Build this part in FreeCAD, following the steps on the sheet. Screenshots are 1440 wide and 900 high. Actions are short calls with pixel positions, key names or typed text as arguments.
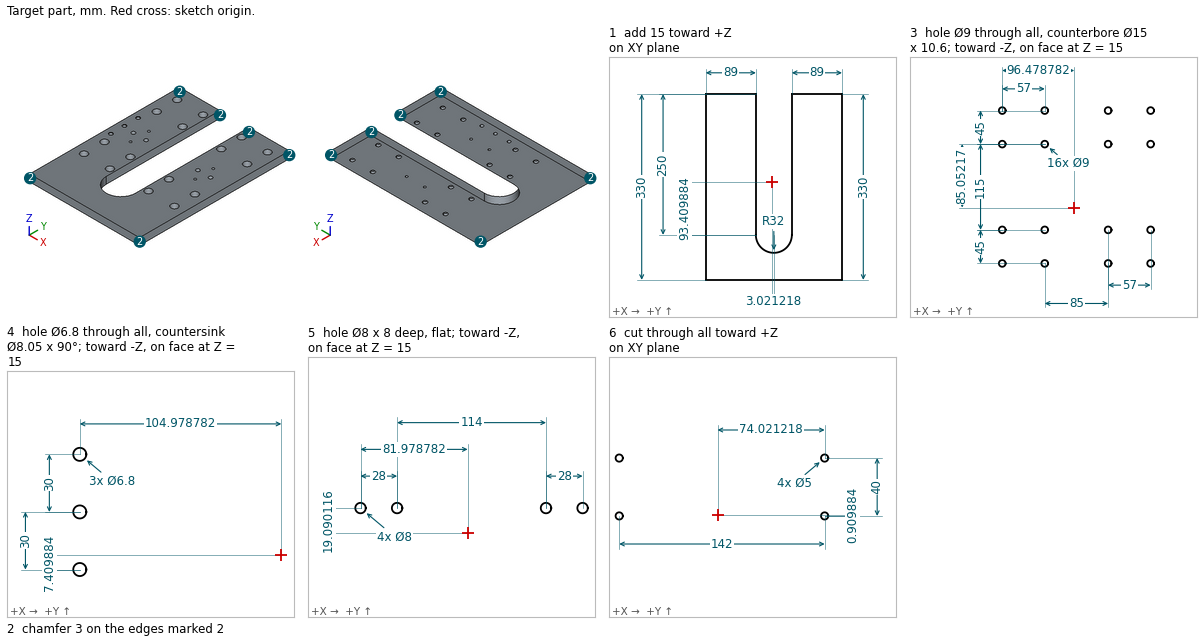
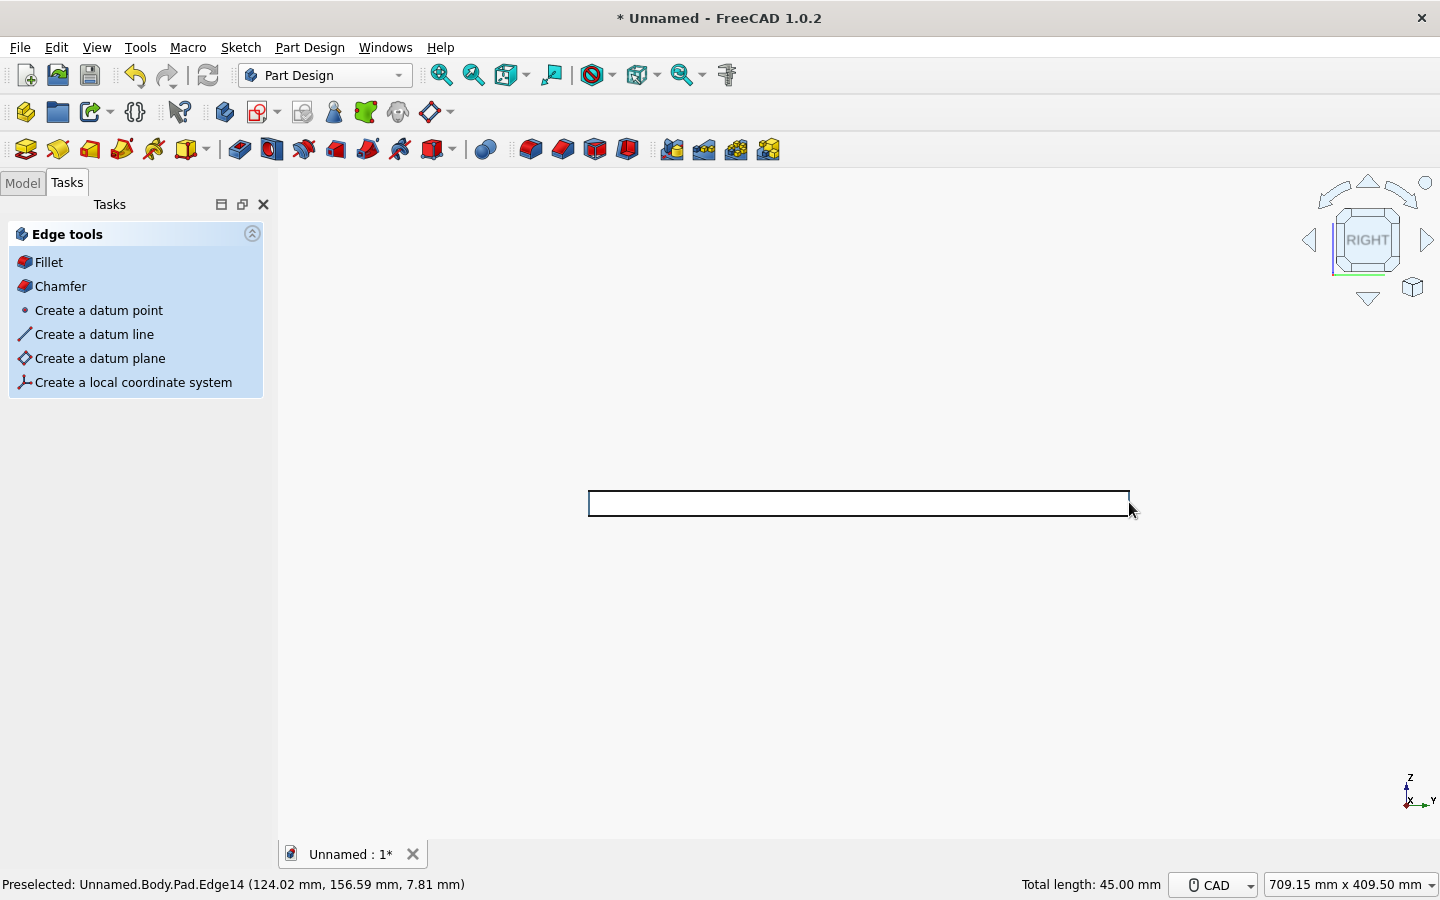
key(5)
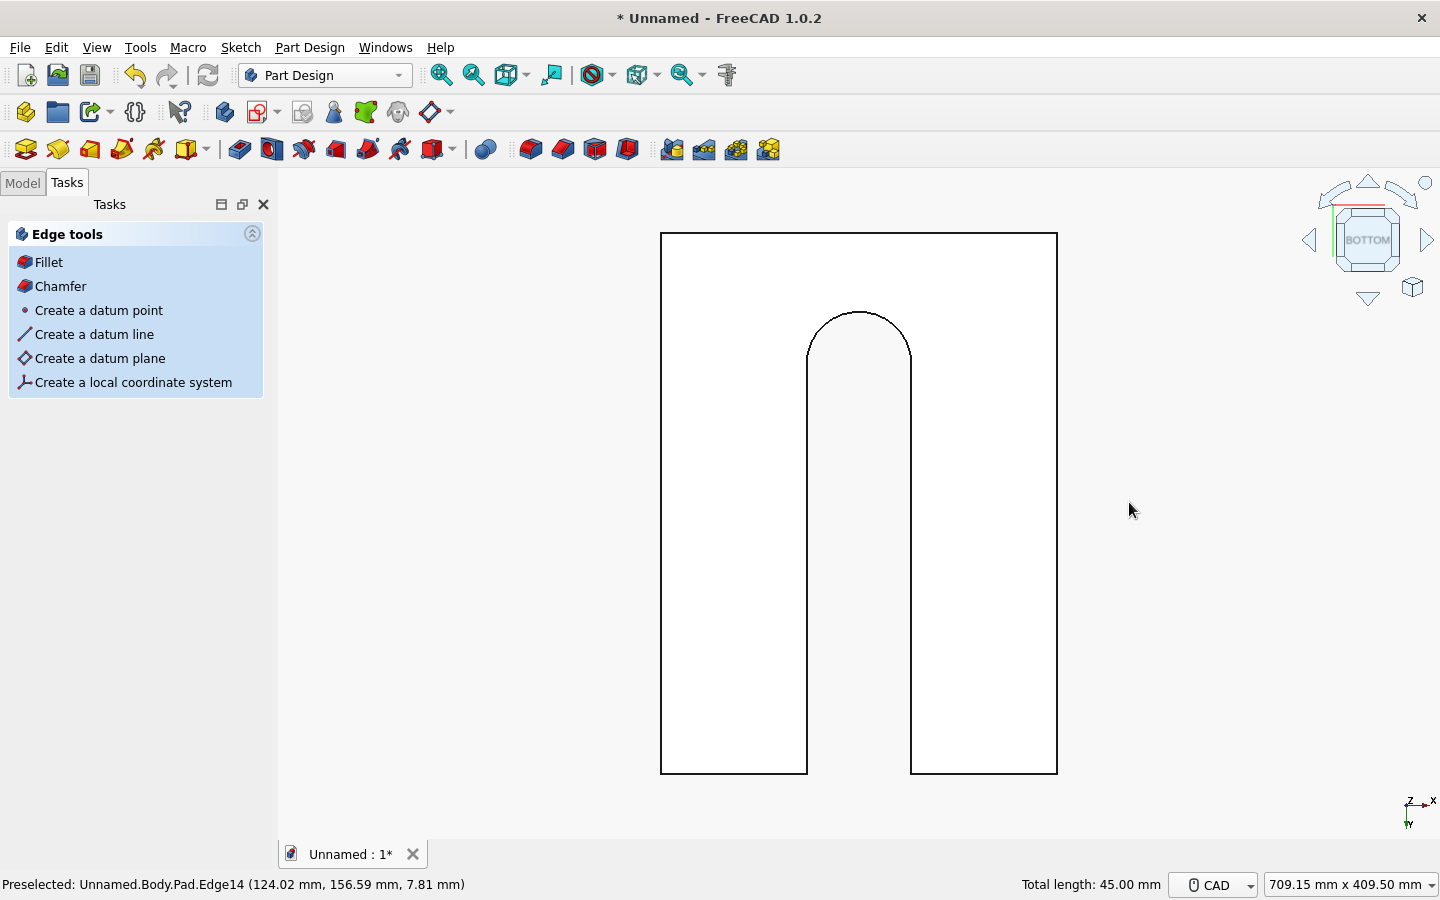
key(4)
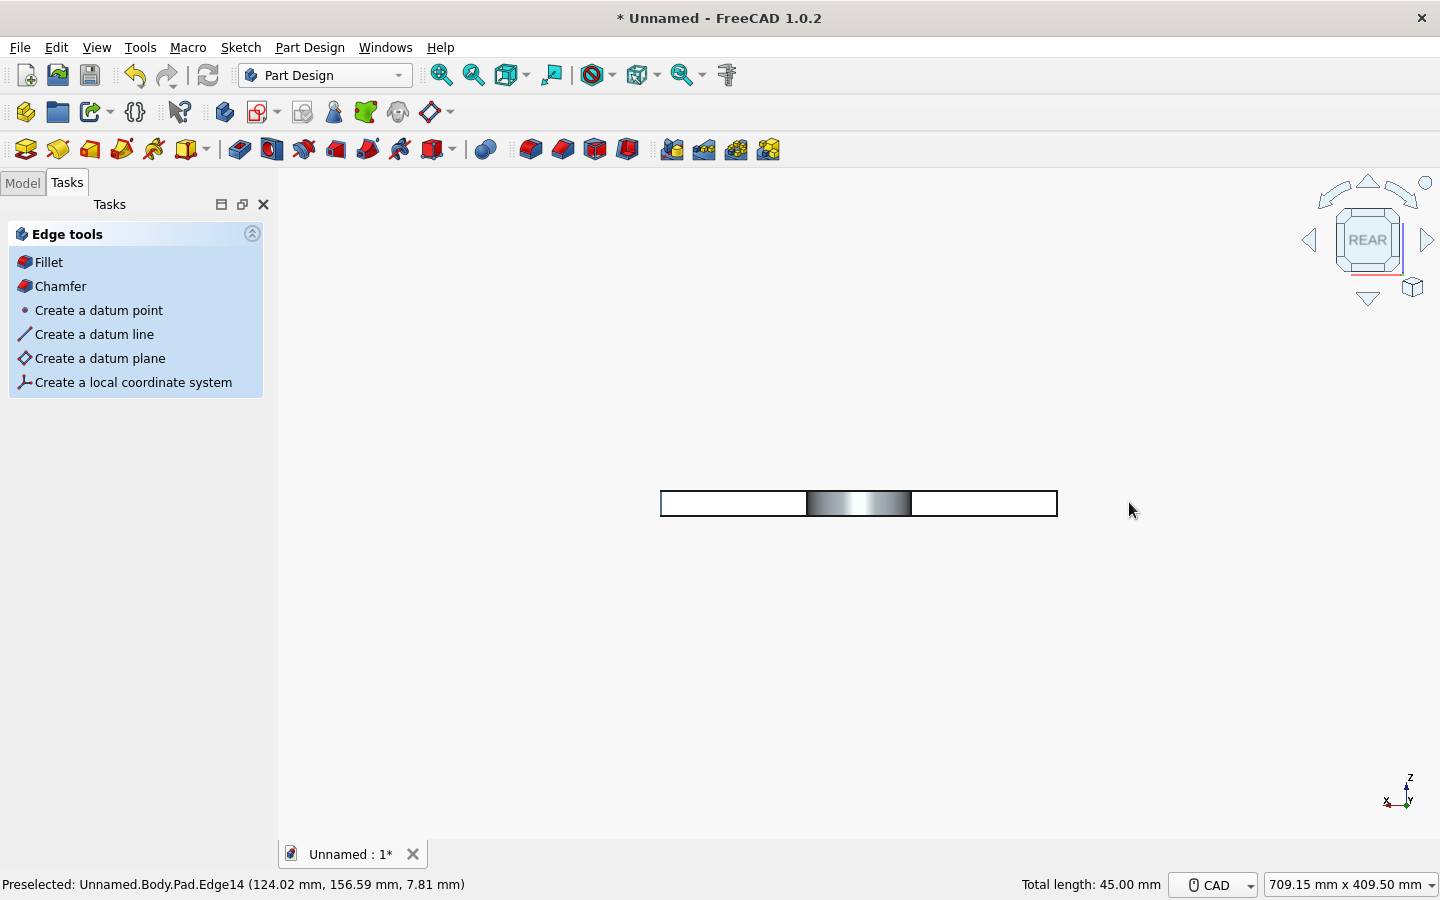
click(442, 76)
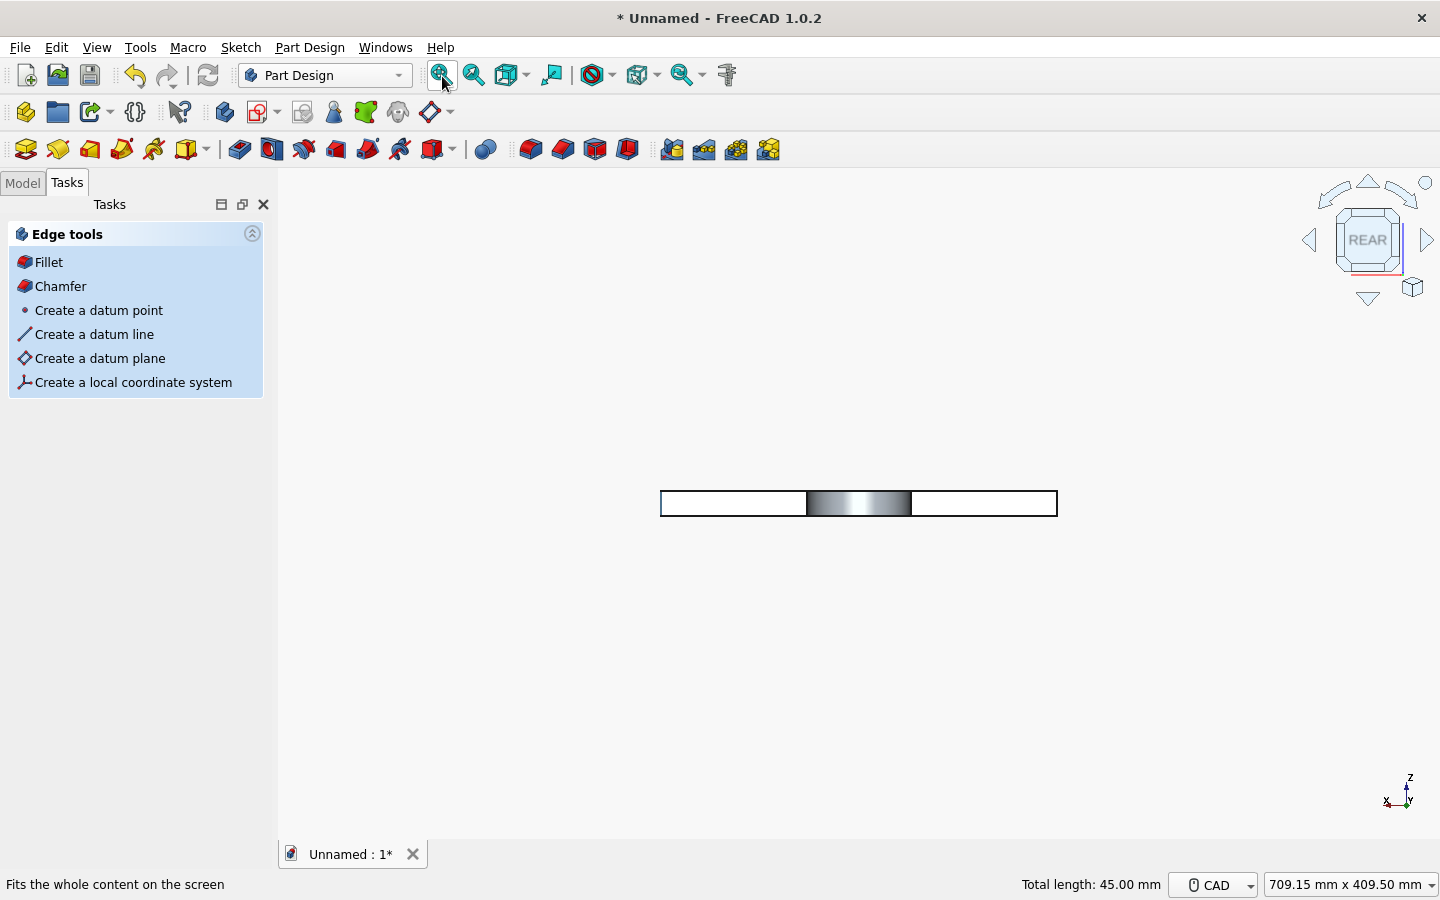
click(1057, 503, ctrl)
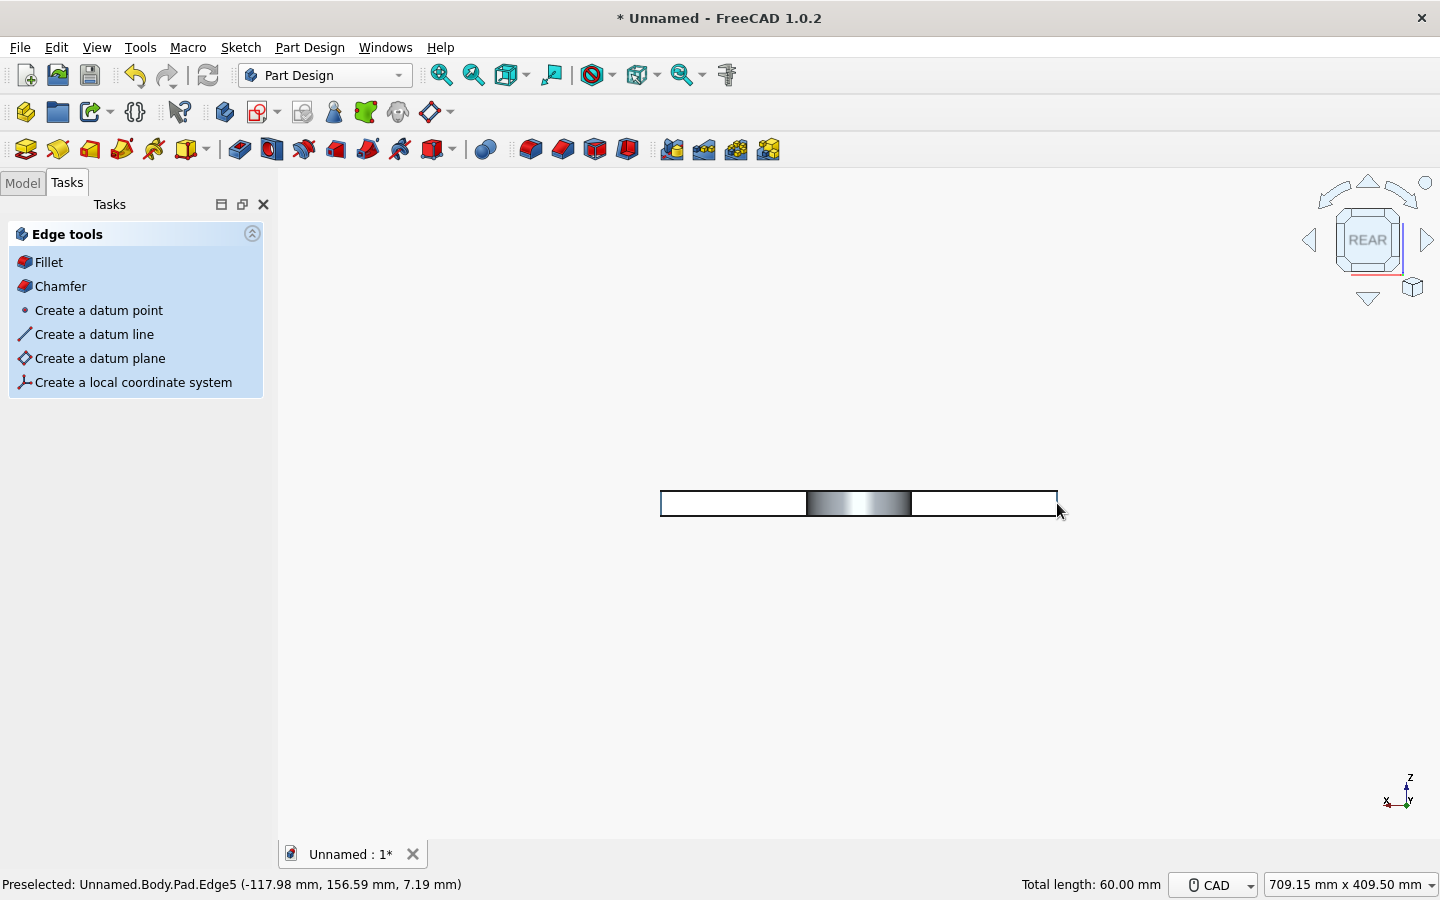
click(911, 503, ctrl)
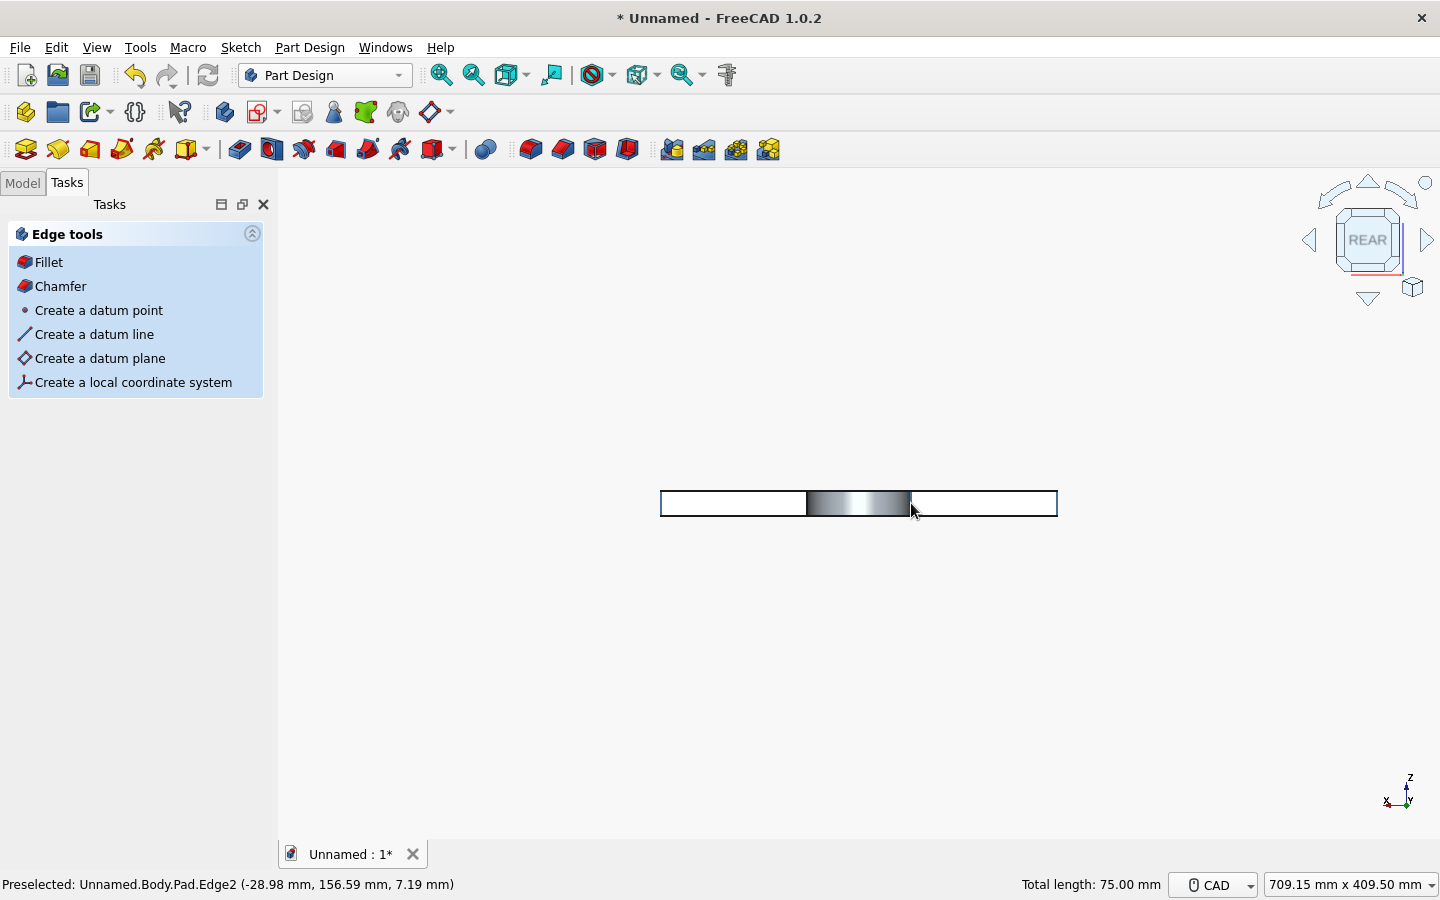
click(807, 503, ctrl)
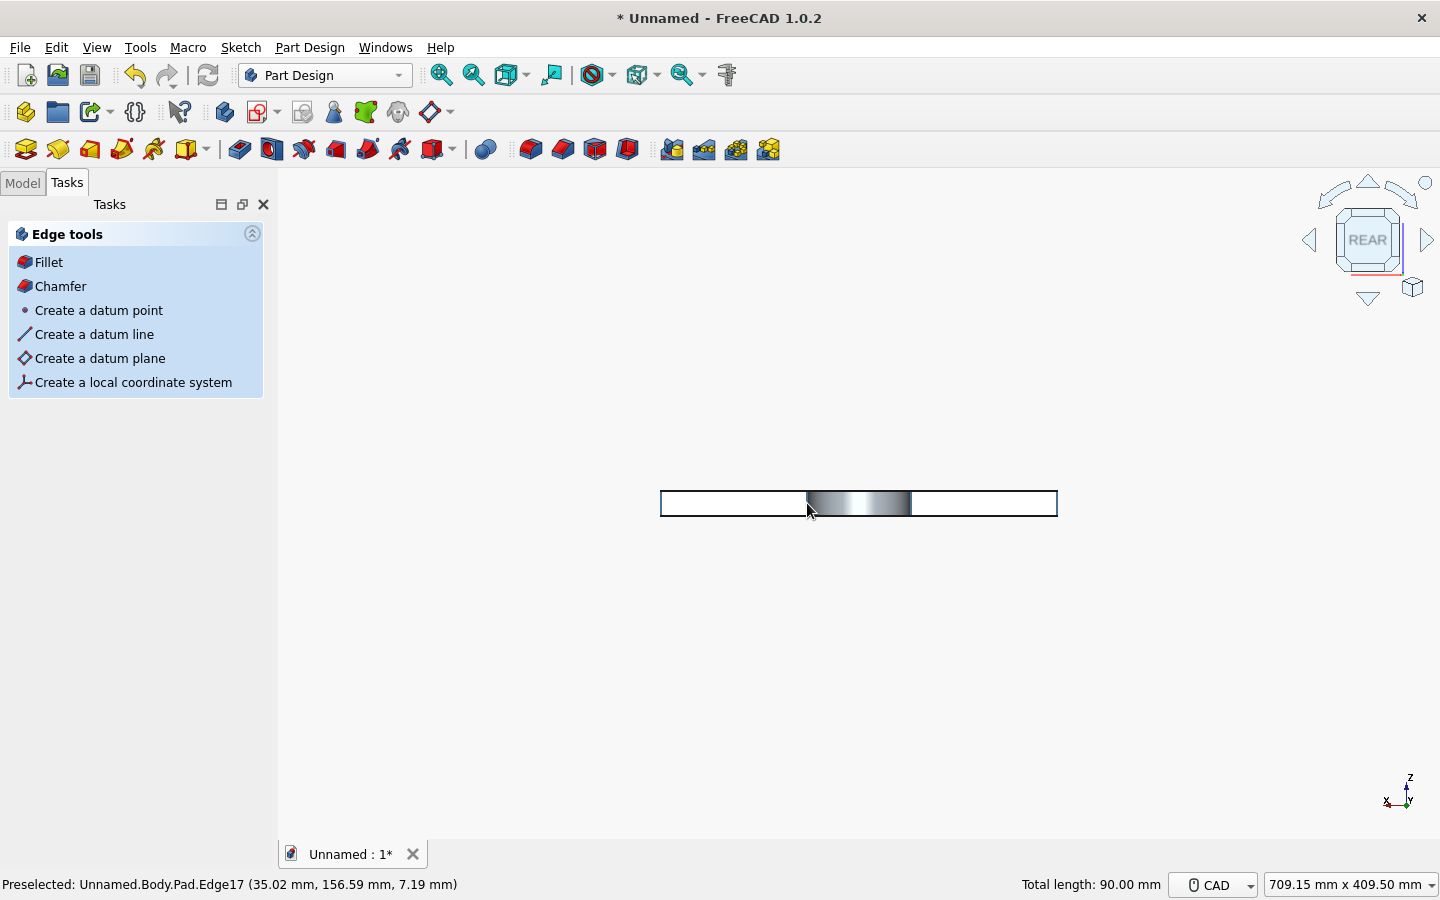
click(564, 150)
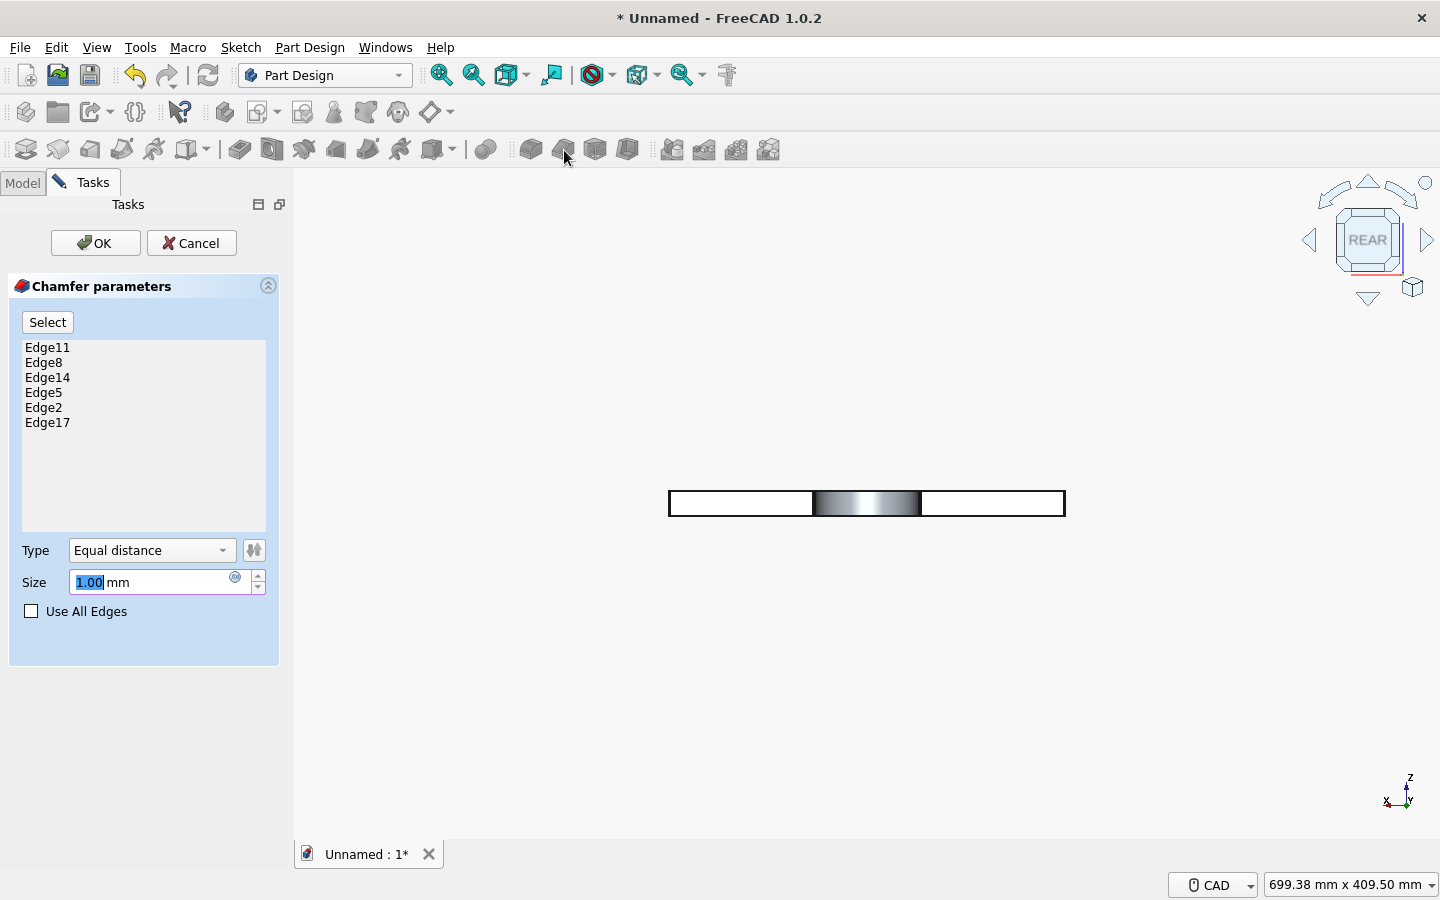
text(3)
key(Tab)